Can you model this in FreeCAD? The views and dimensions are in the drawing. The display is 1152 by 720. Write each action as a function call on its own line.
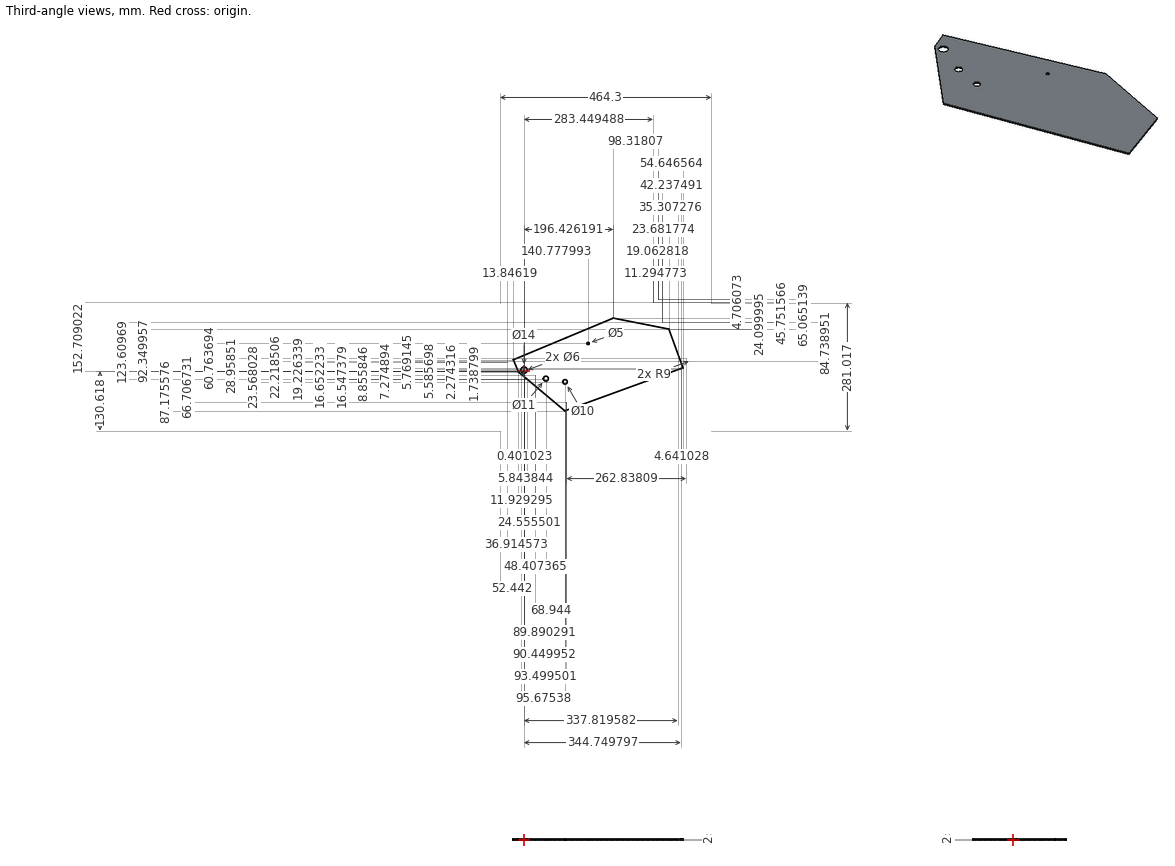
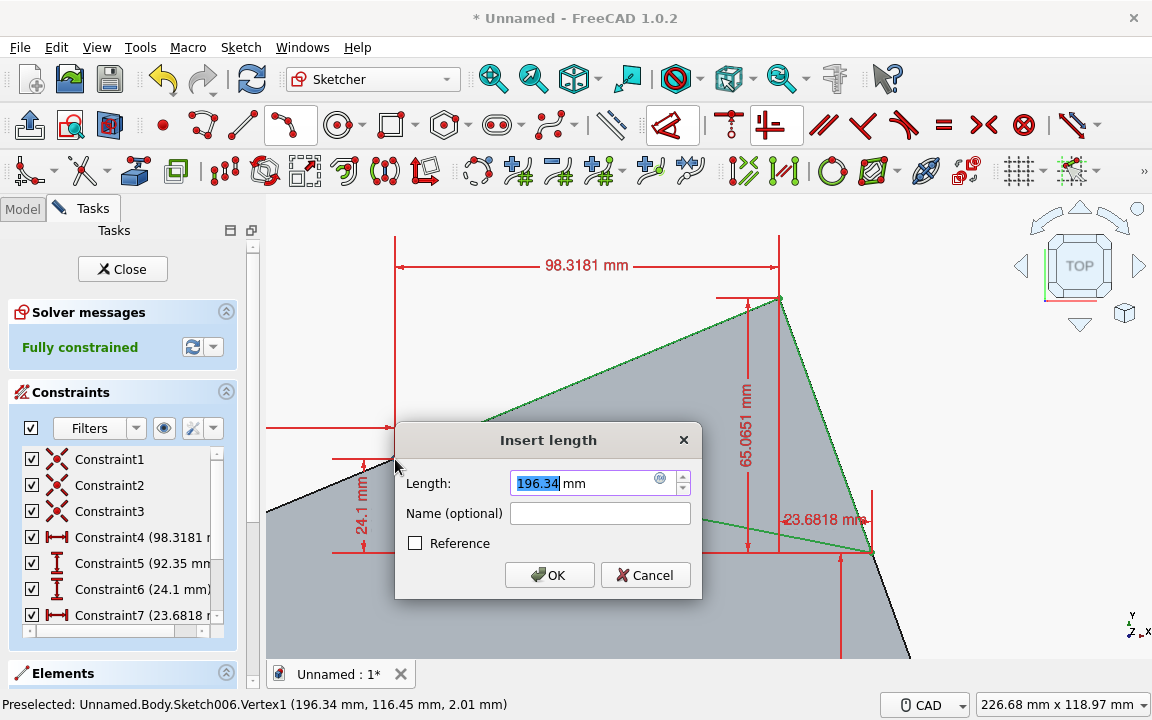
text(196.426191)
key(Return)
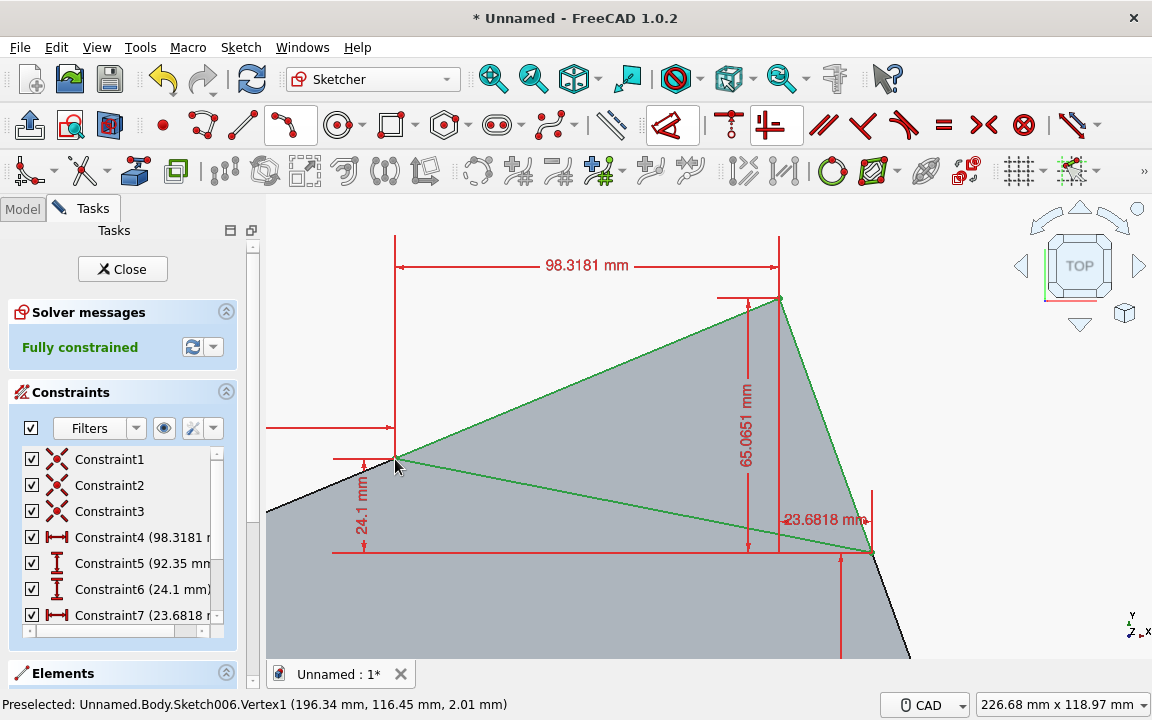
click(123, 269)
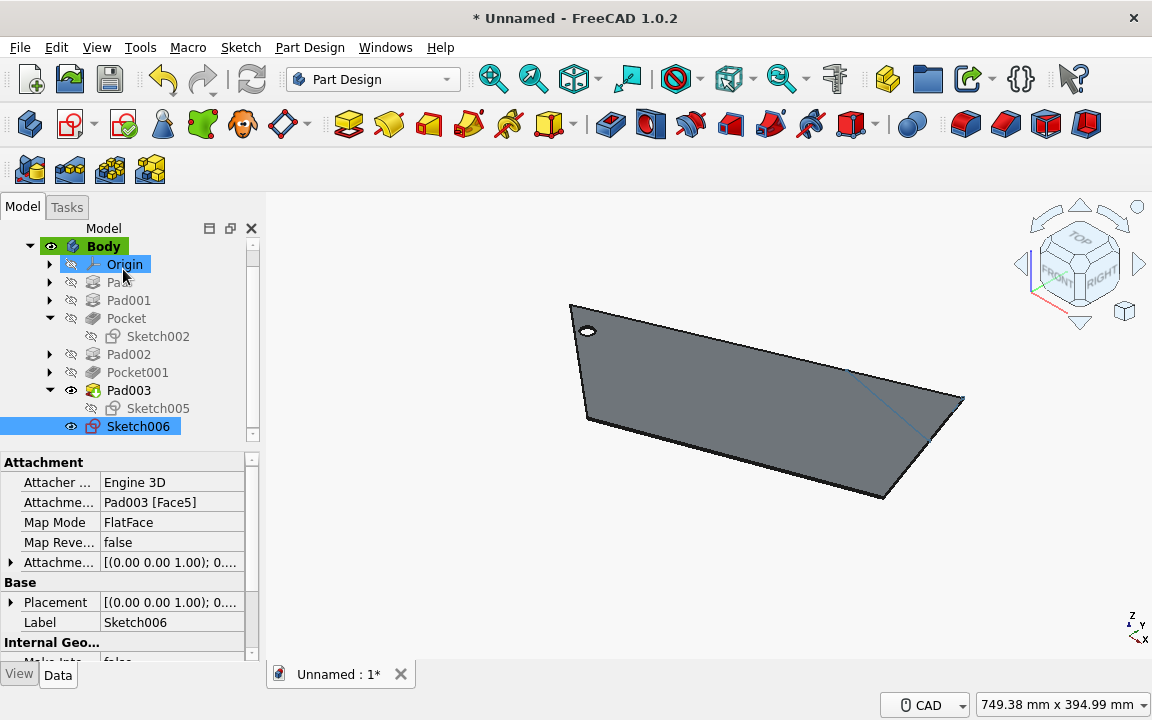
click(612, 124)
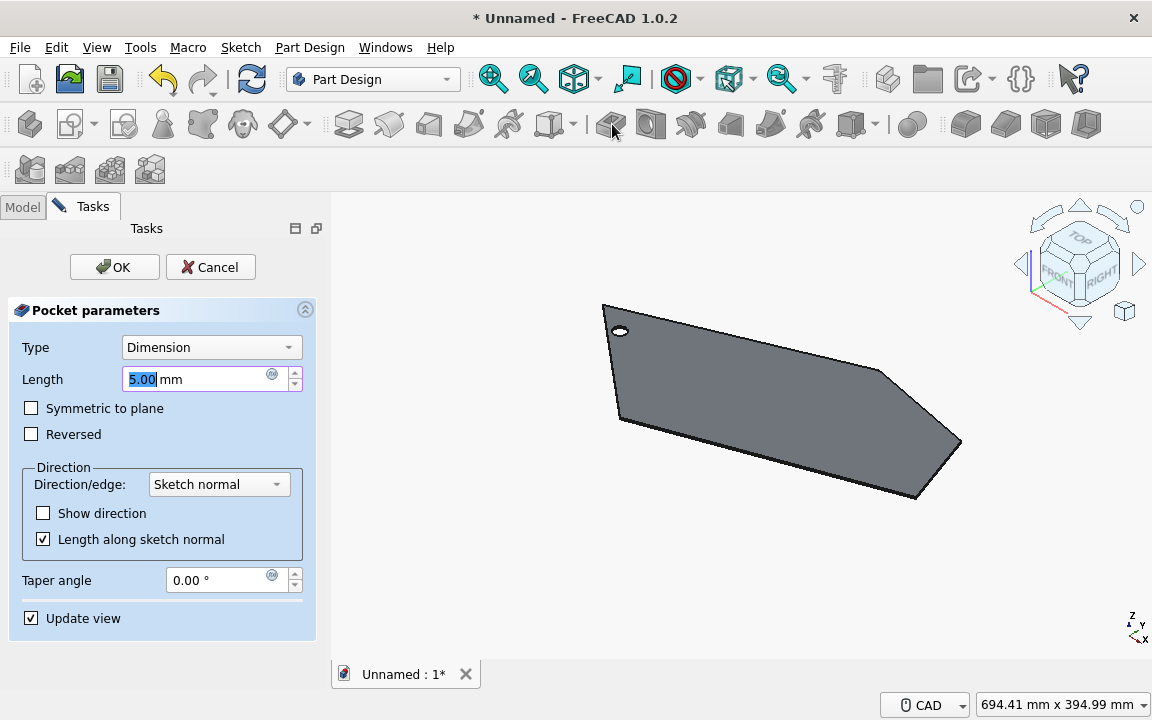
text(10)
key(Tab)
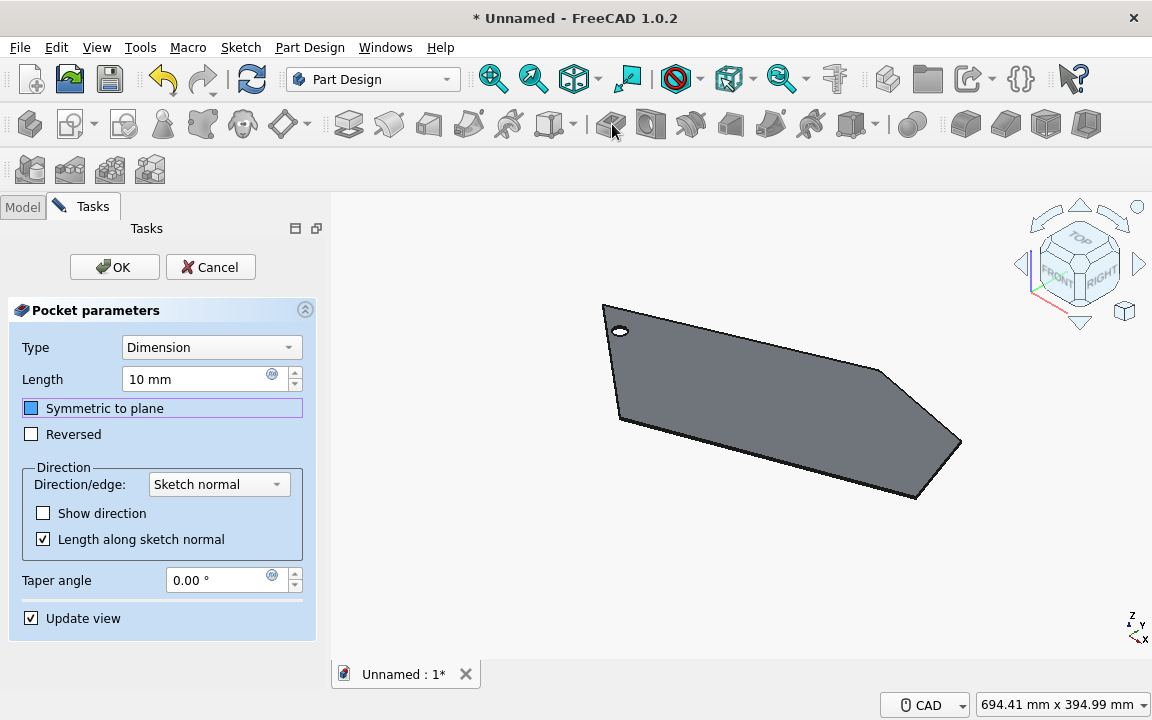
click(115, 267)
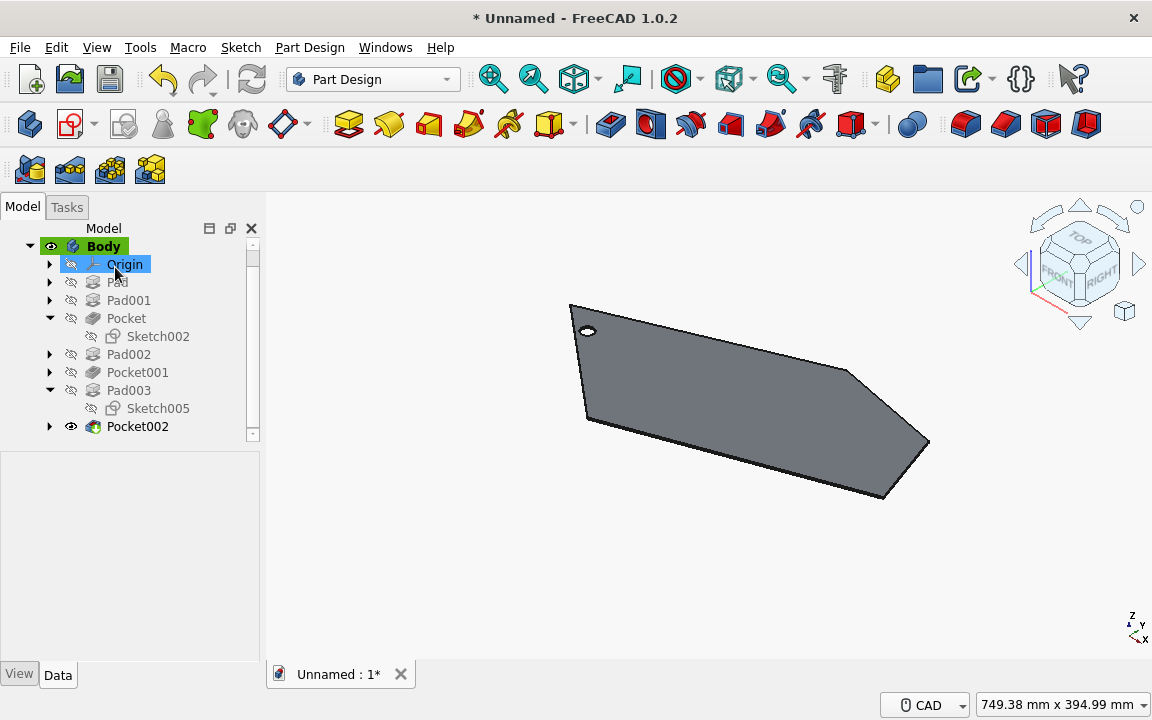
key(5)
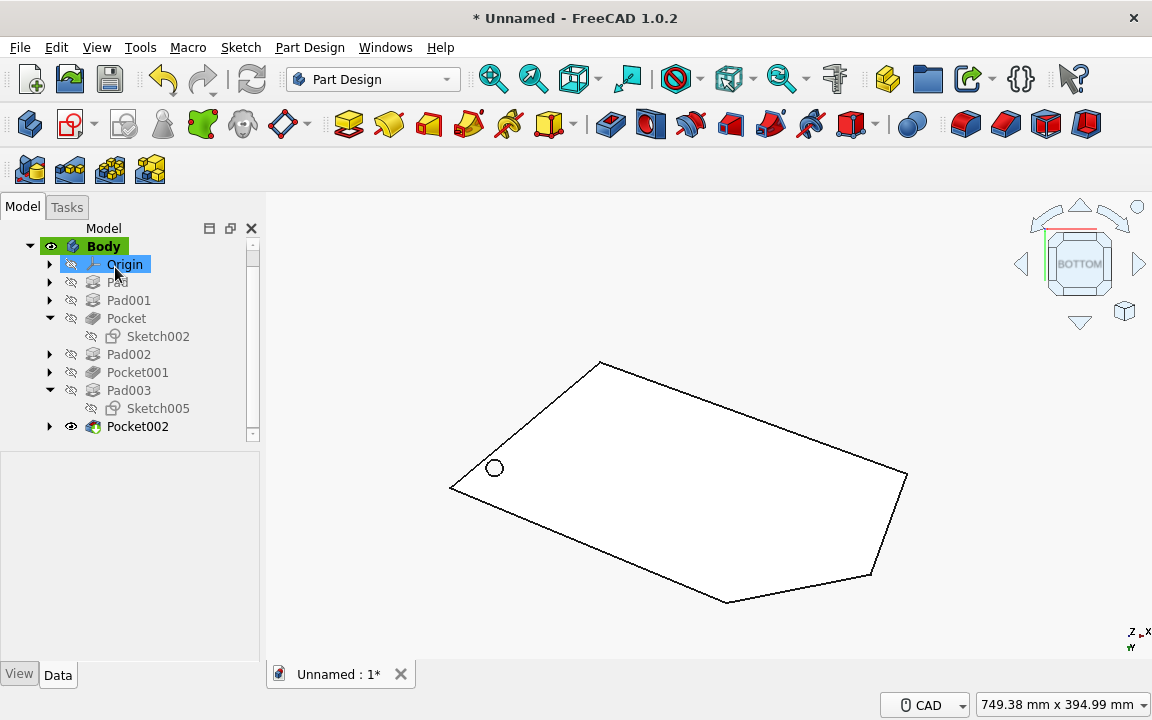
click(679, 482)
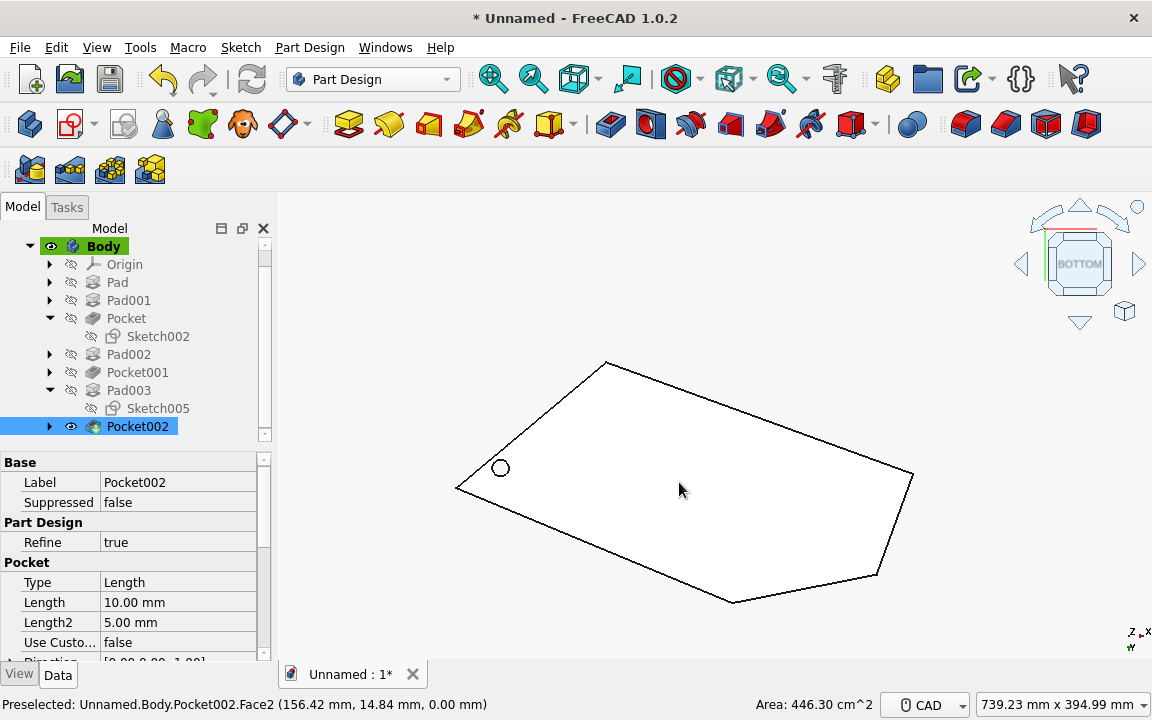
click(70, 124)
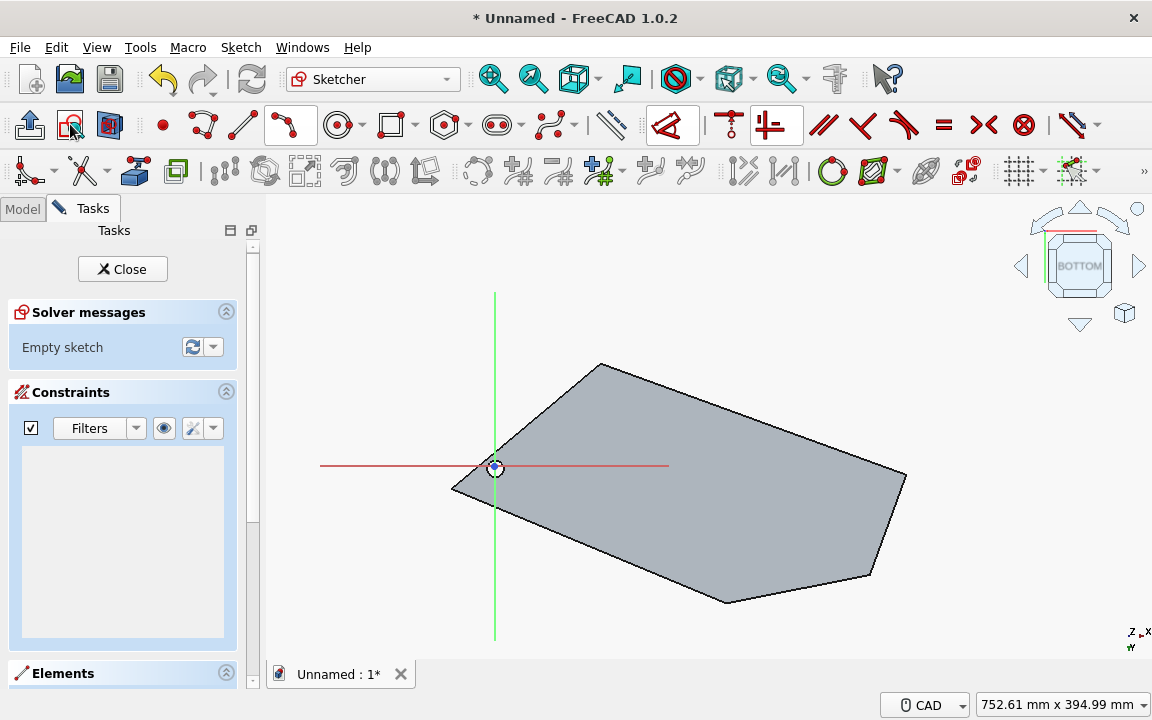
scroll(452, 487, up, 11)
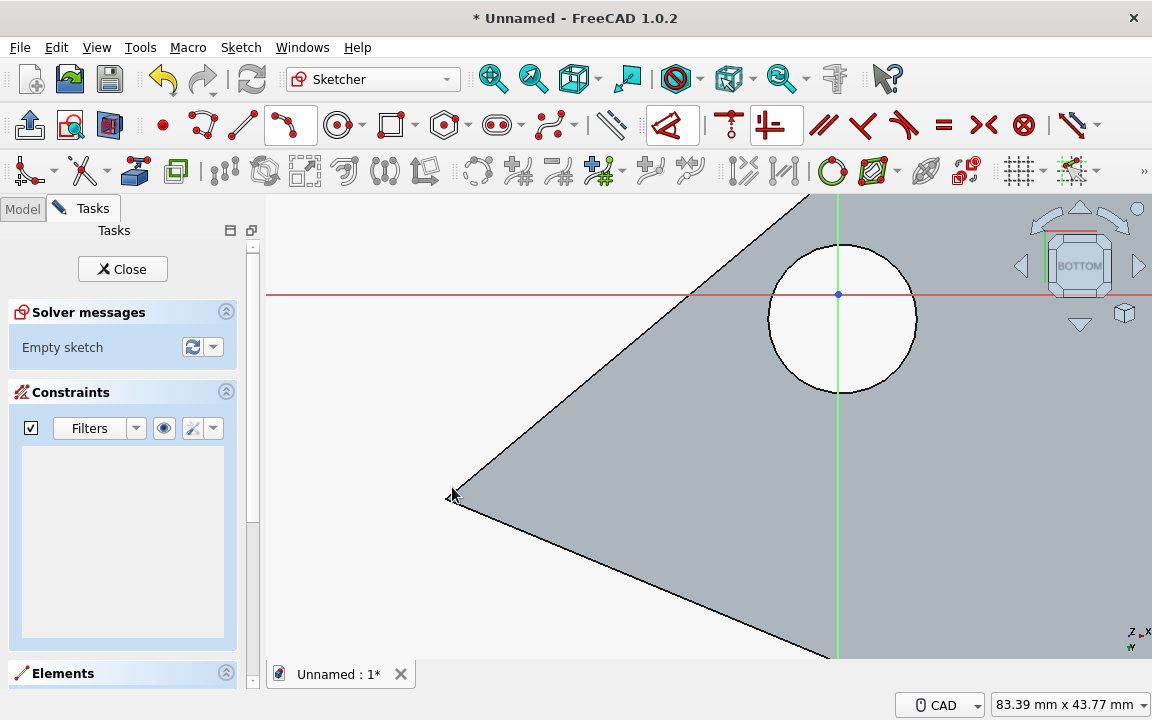
click(204, 126)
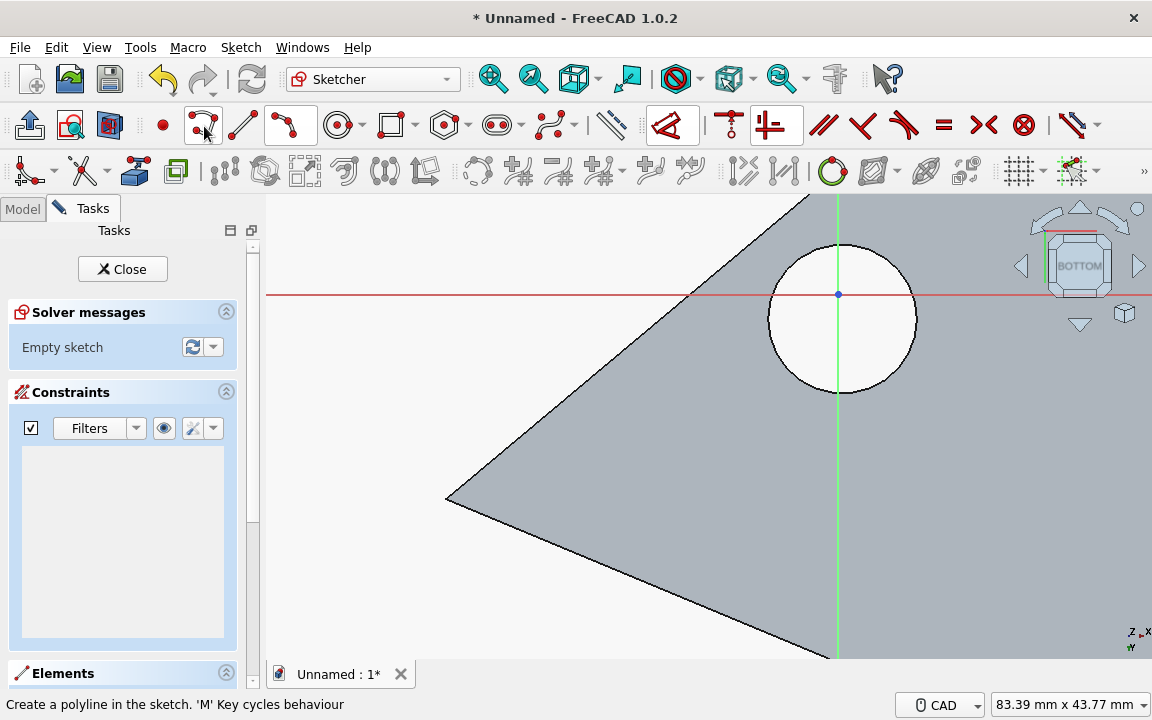
click(712, 276)
click(446, 499)
click(593, 560)
click(712, 277)
key(Escape)
key(Escape)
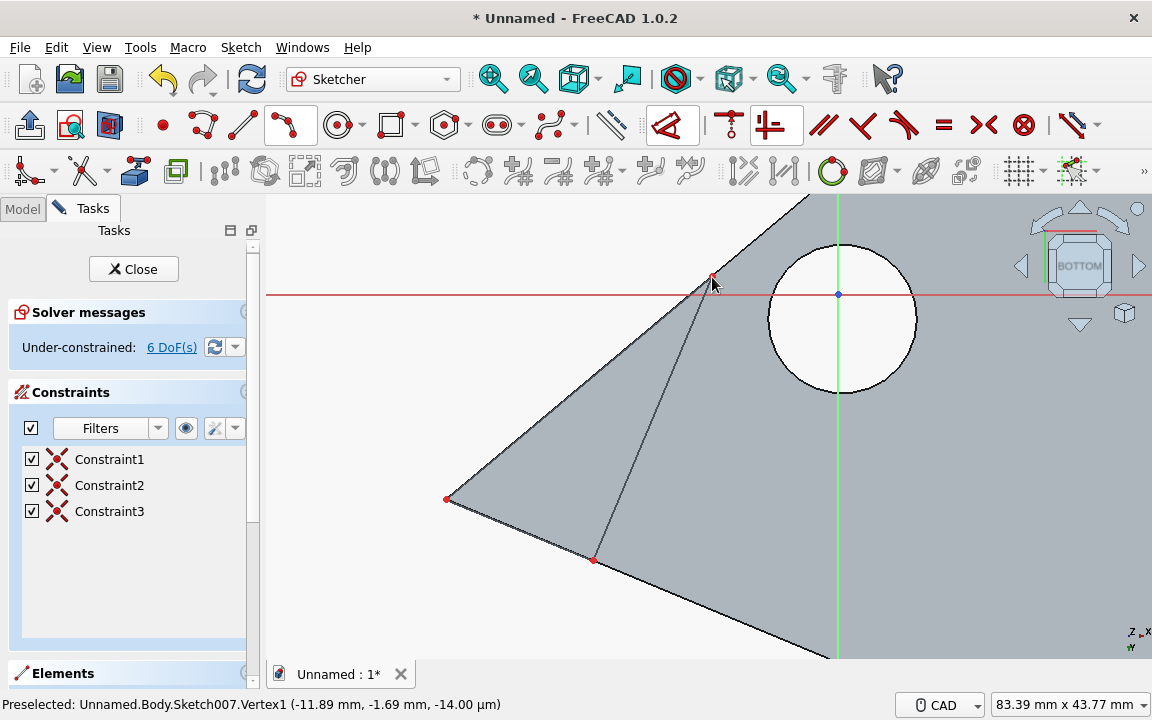
scroll(712, 277, up, 4)